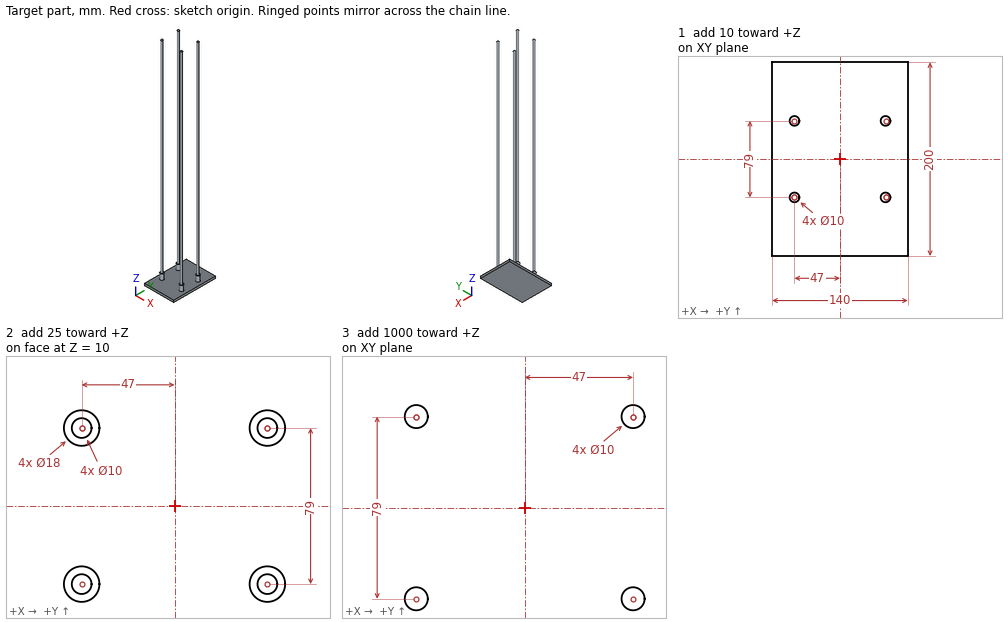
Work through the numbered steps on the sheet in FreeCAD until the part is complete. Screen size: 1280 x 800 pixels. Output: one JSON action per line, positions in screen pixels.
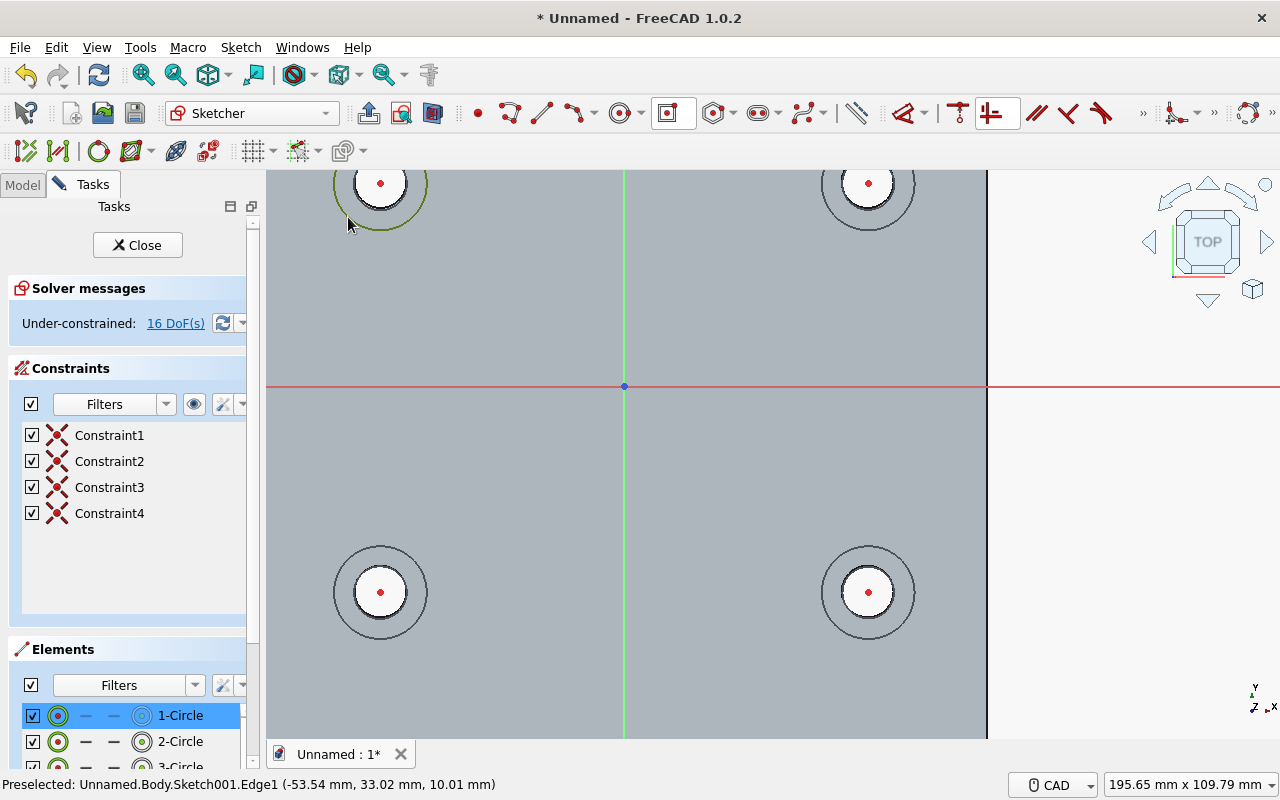
{"action": "left_click", "coordinate": [835, 217]}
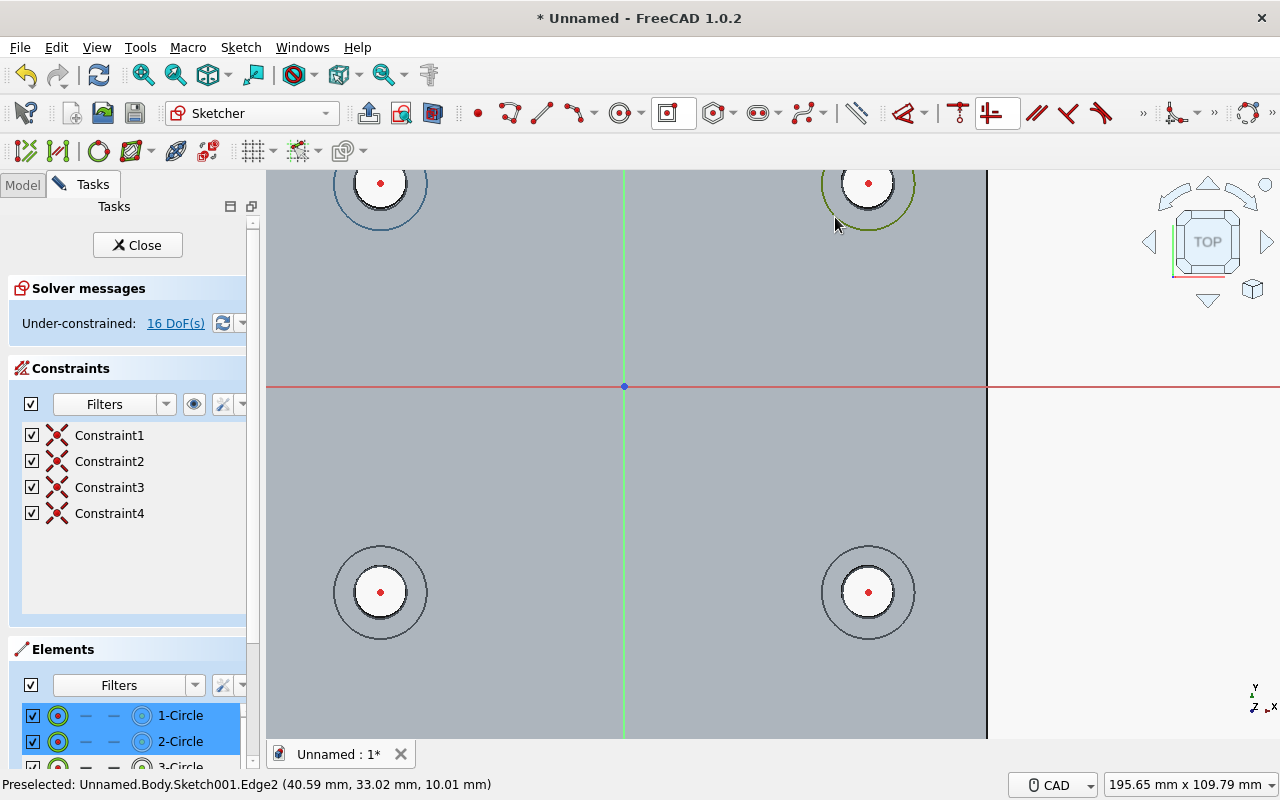
{"action": "left_click", "coordinate": [901, 560]}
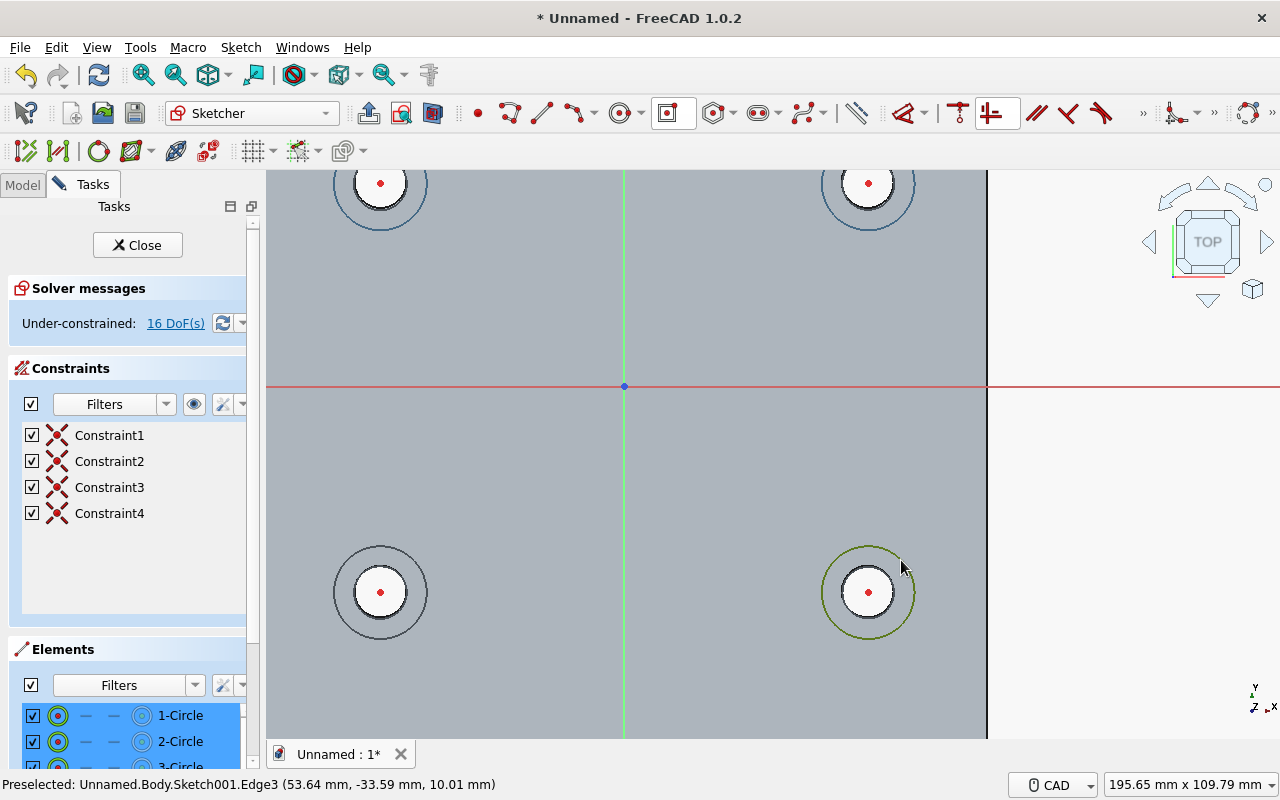
{"action": "left_click", "coordinate": [413, 560]}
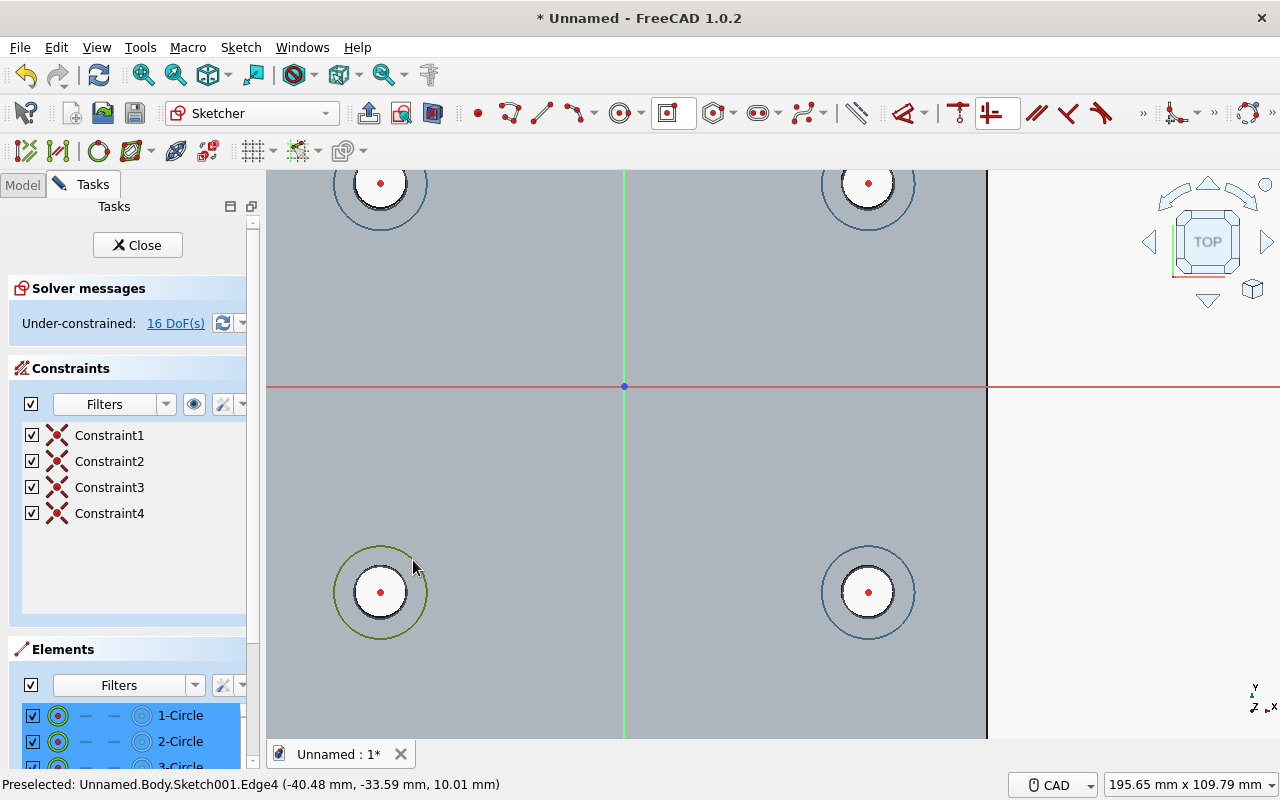
{"action": "key", "text": "e"}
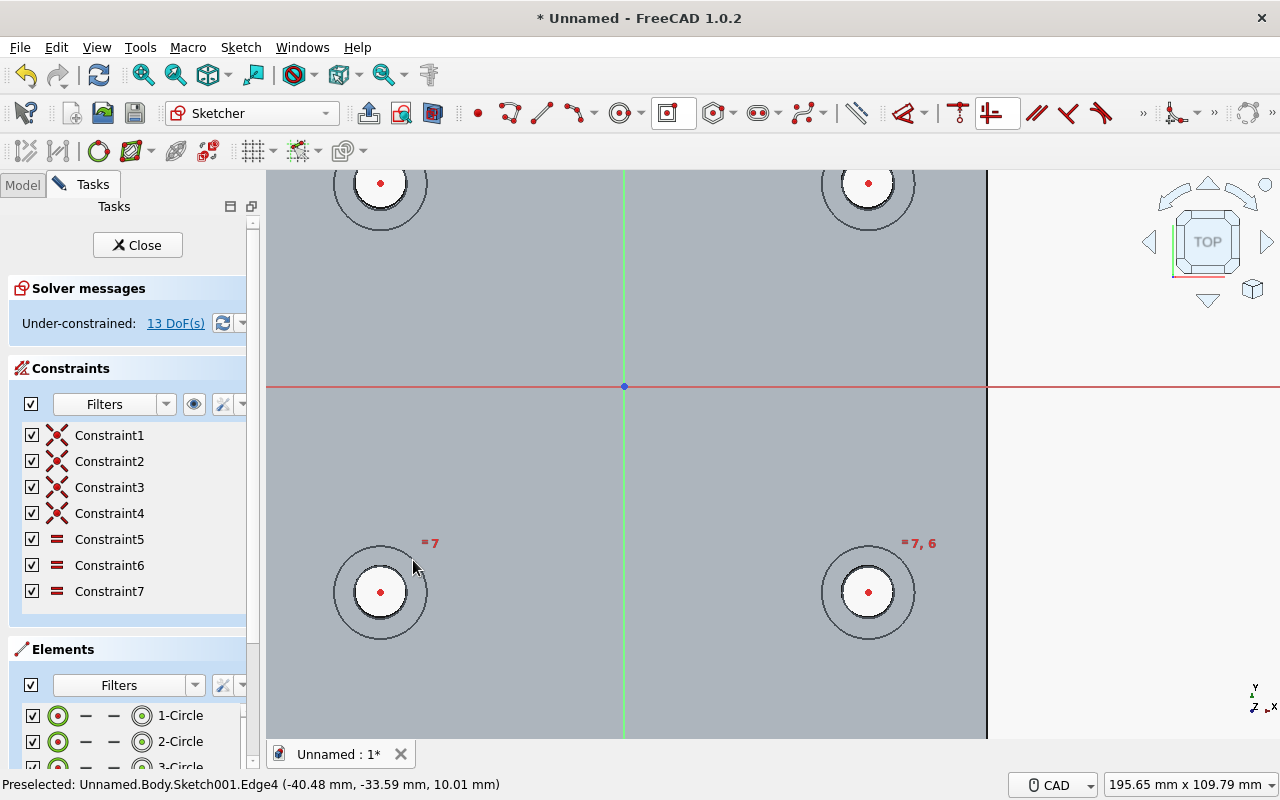
{"action": "left_click", "coordinate": [362, 203]}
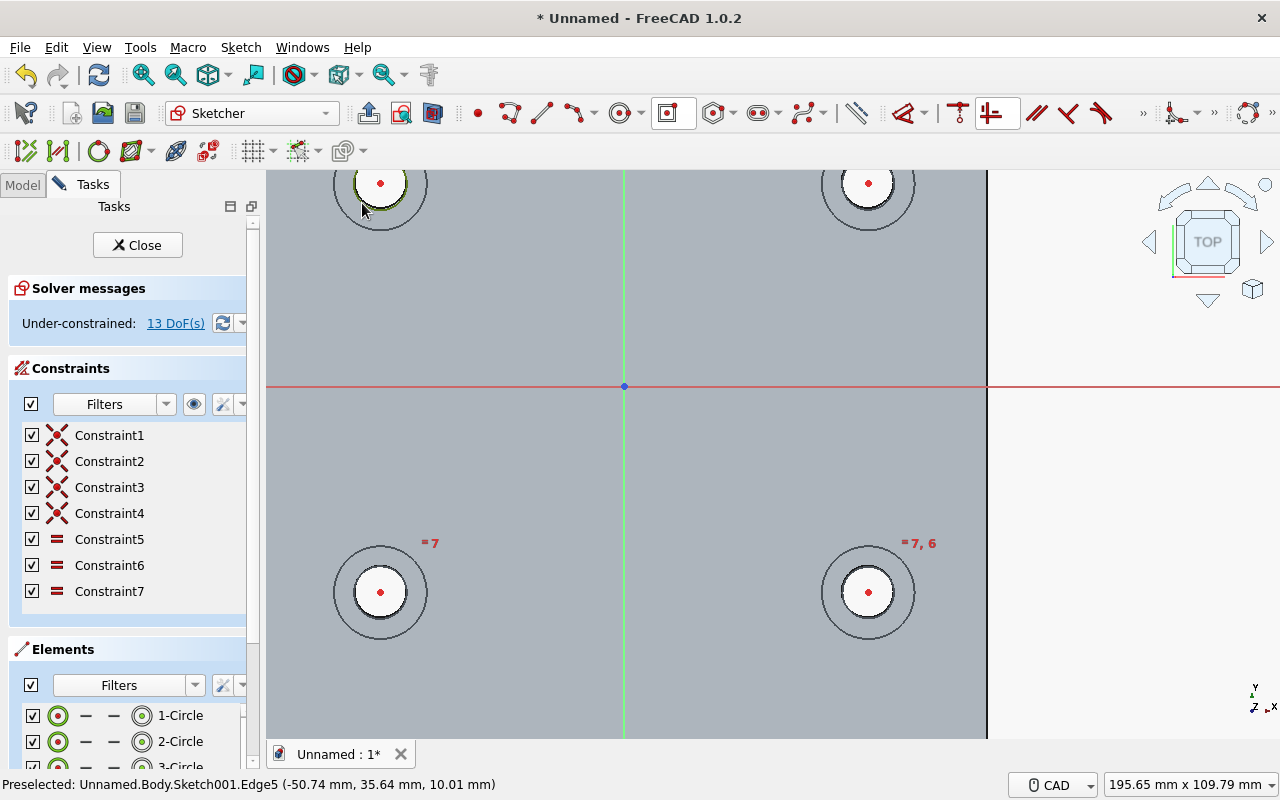
{"action": "left_click", "coordinate": [850, 202]}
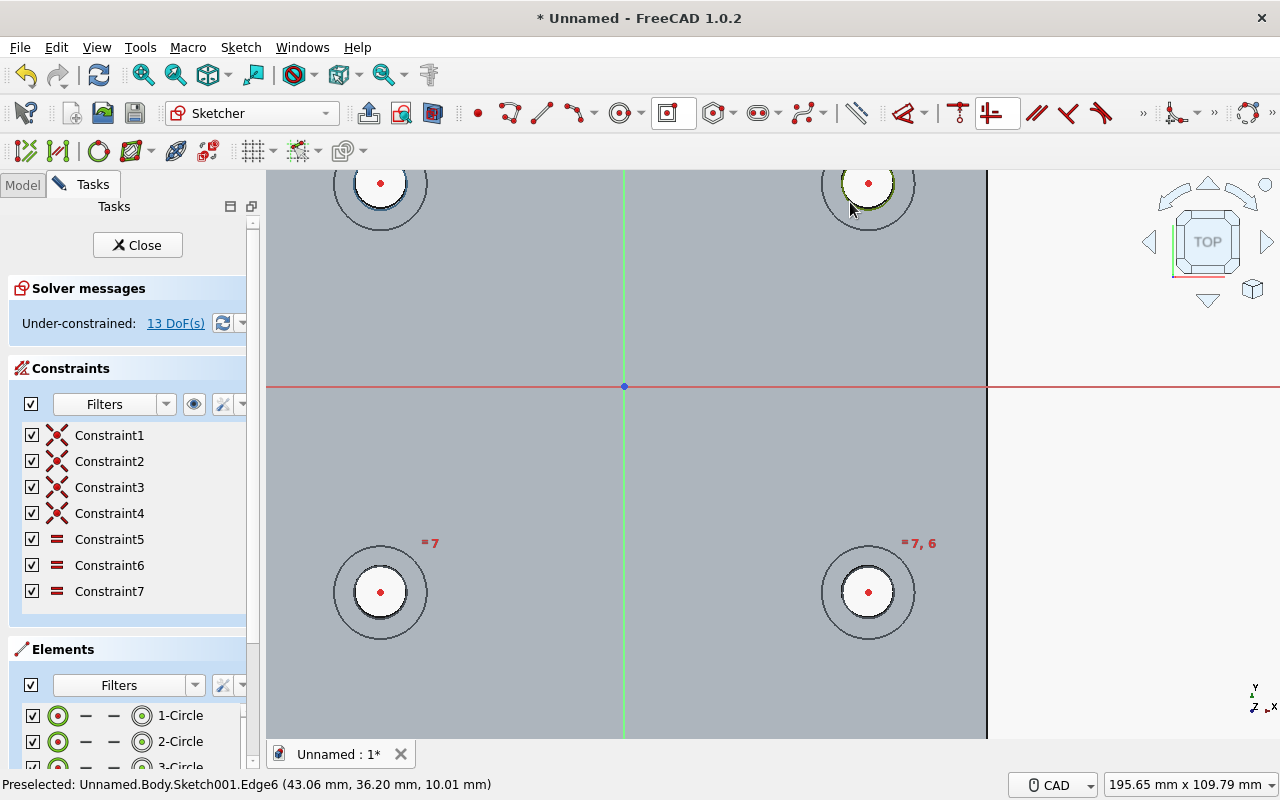
{"action": "left_click", "coordinate": [886, 574]}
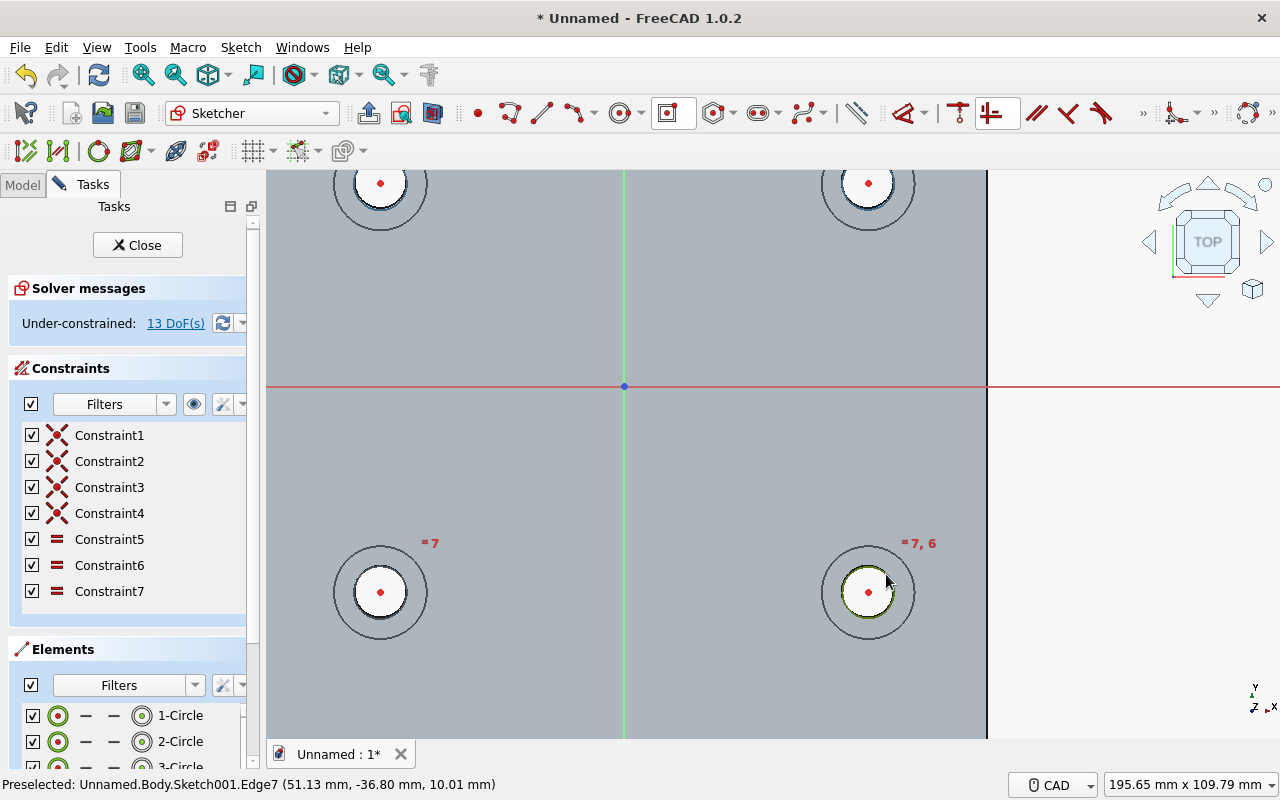
{"action": "left_click", "coordinate": [399, 574]}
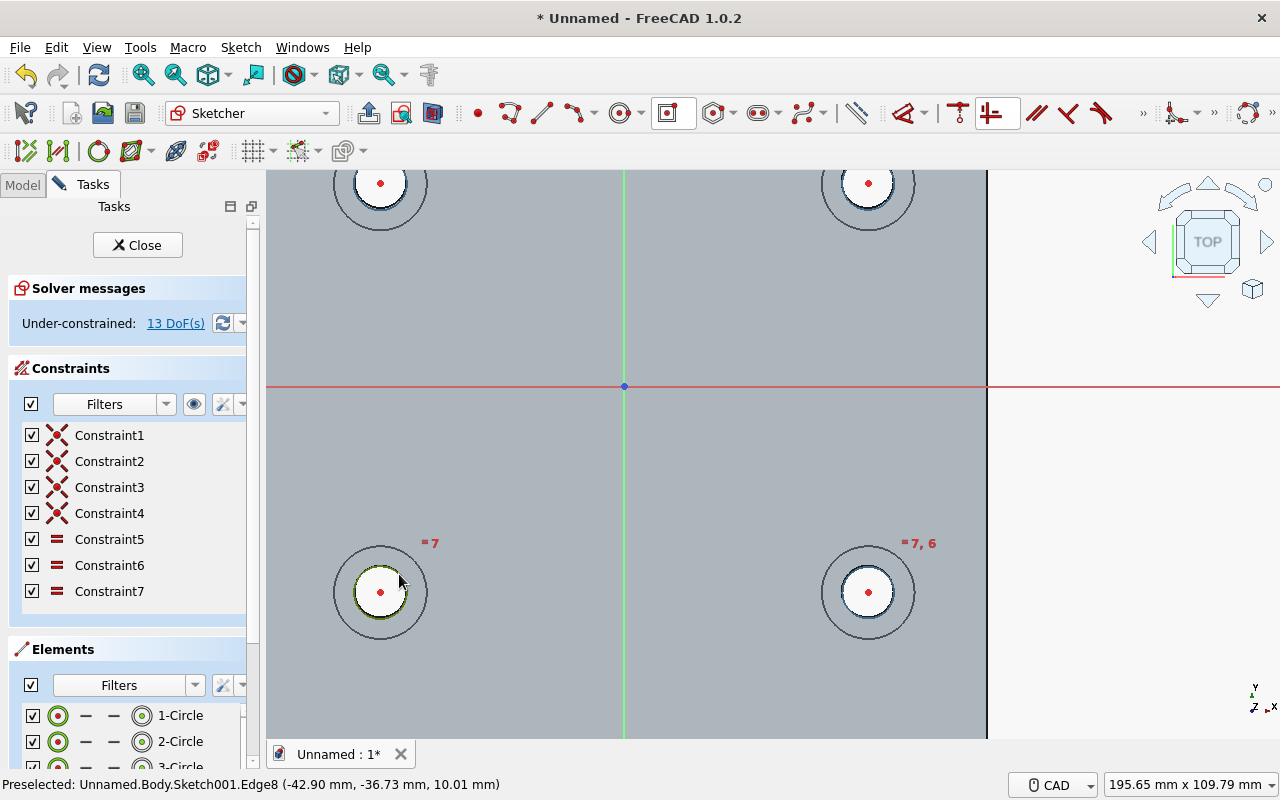
{"action": "key", "text": "e"}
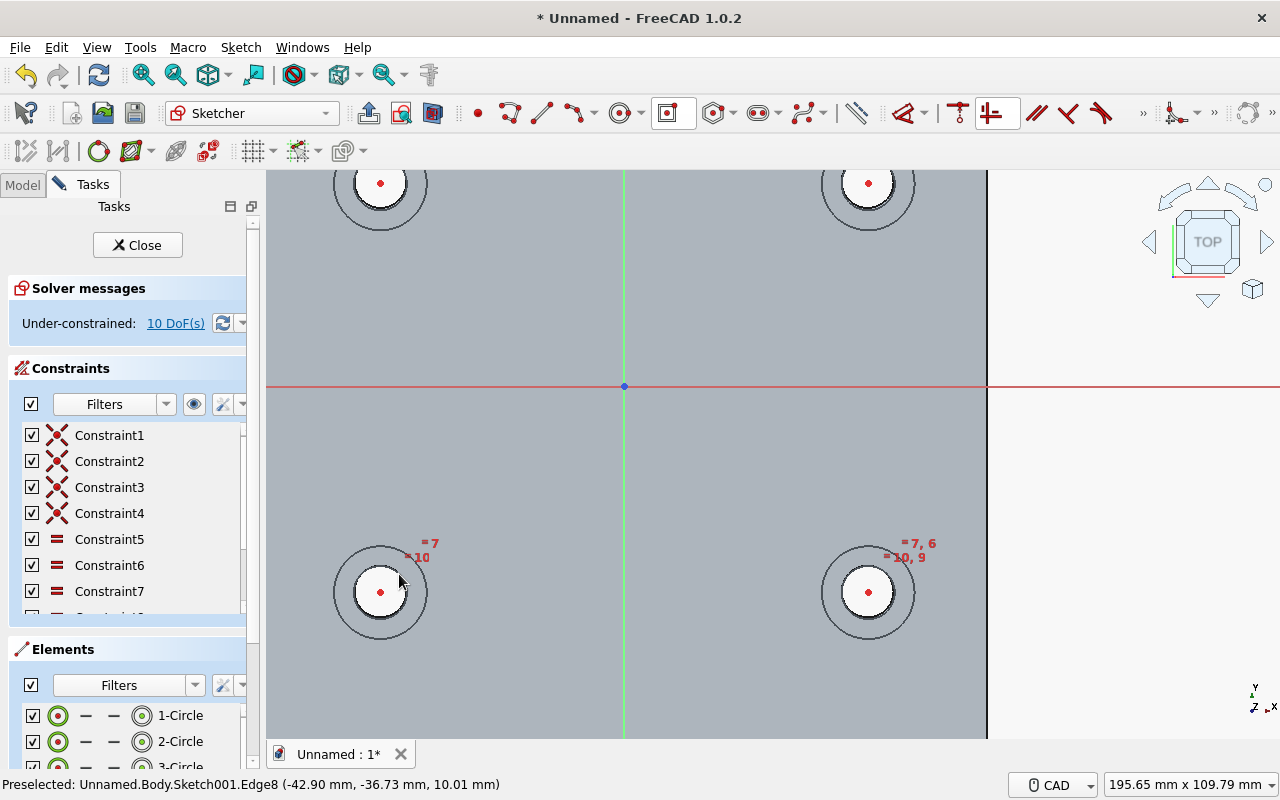
{"action": "scroll", "coordinate": [868, 592], "scroll_direction": "down", "scroll_amount": 2}